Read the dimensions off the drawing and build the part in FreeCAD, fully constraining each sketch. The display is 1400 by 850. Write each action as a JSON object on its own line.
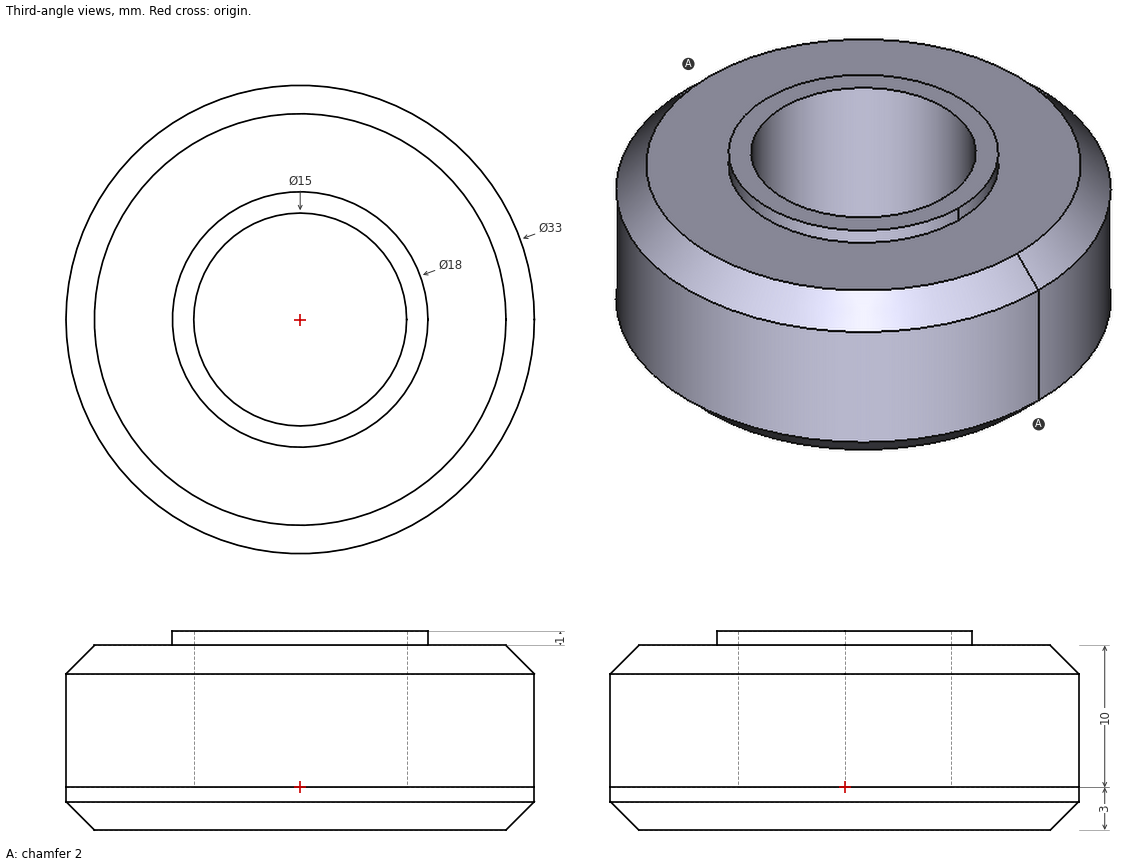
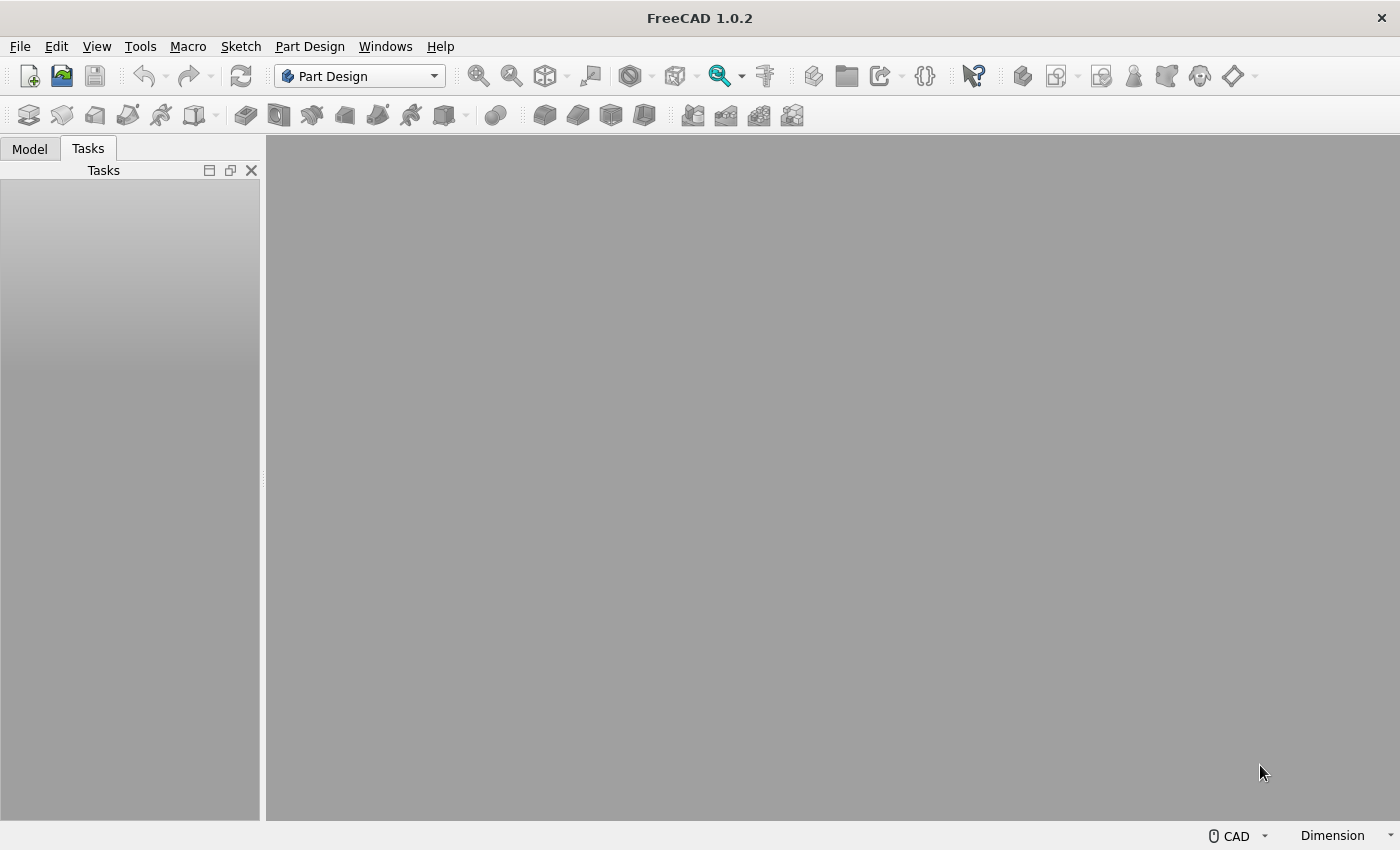
{"action": "key", "text": "ctrl+n"}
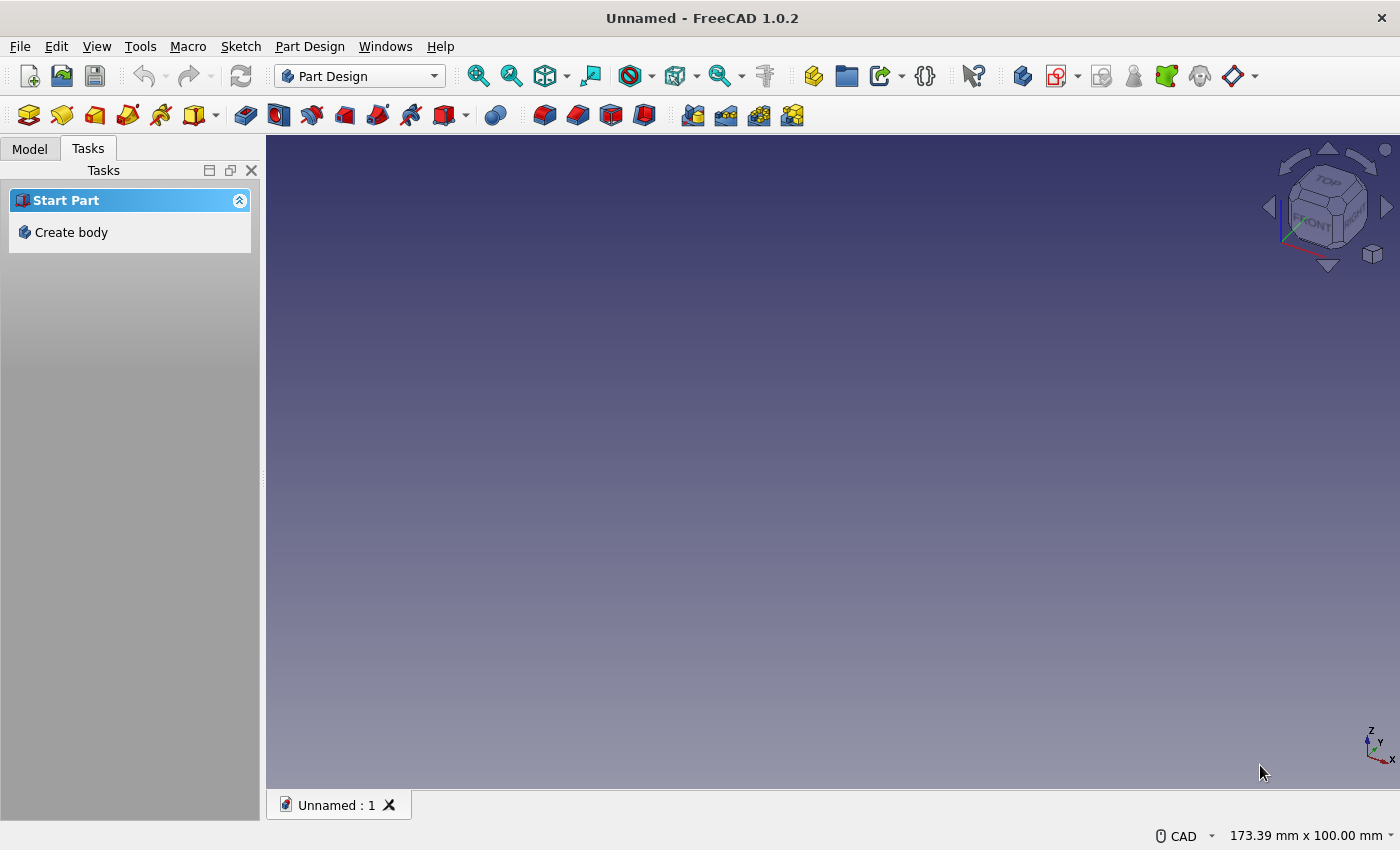
{"action": "left_click", "coordinate": [1056, 76]}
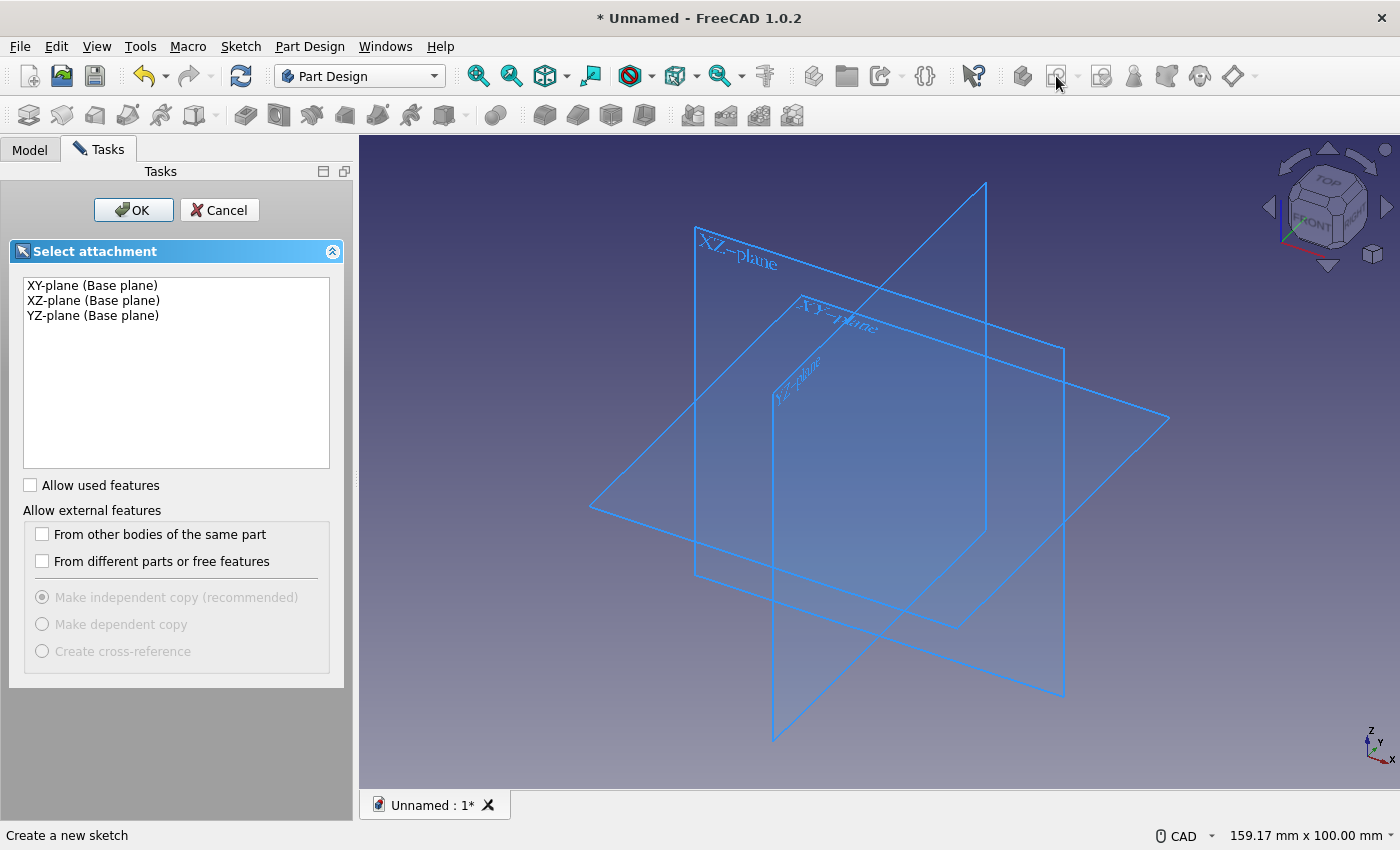
{"action": "left_click", "coordinate": [84, 286]}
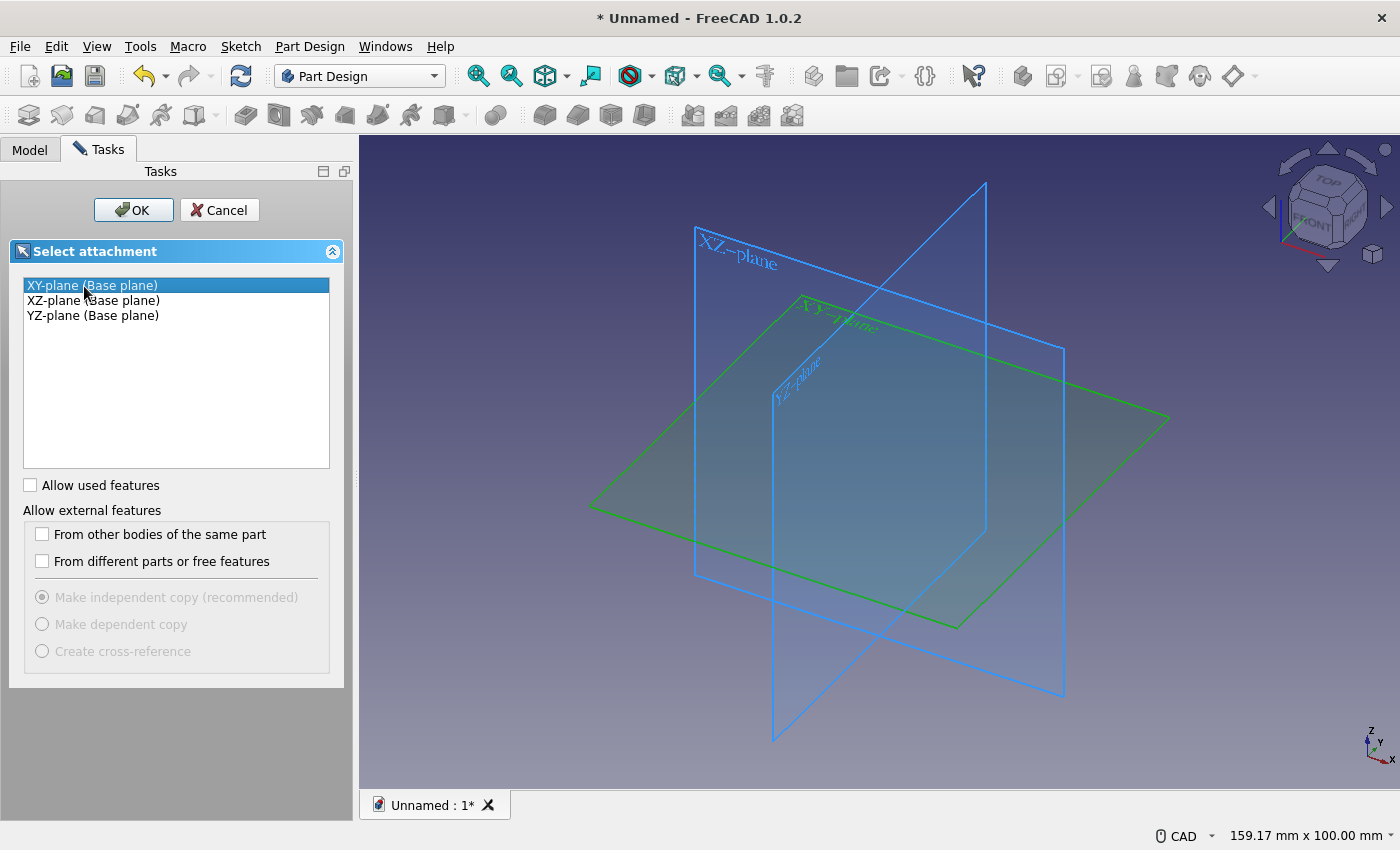
{"action": "left_click", "coordinate": [134, 210]}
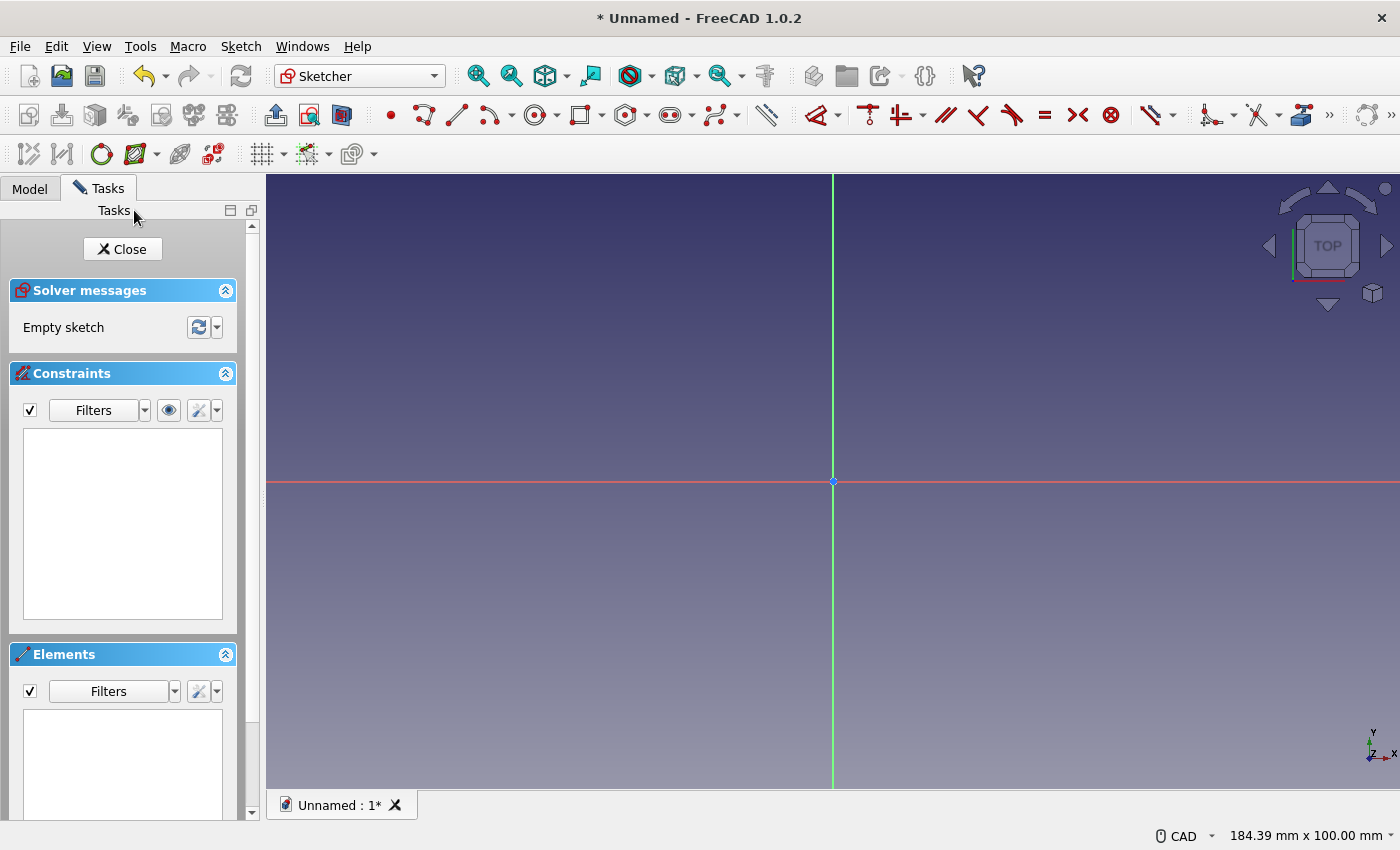
{"action": "scroll", "coordinate": [916, 481], "scroll_direction": "up", "scroll_amount": 3}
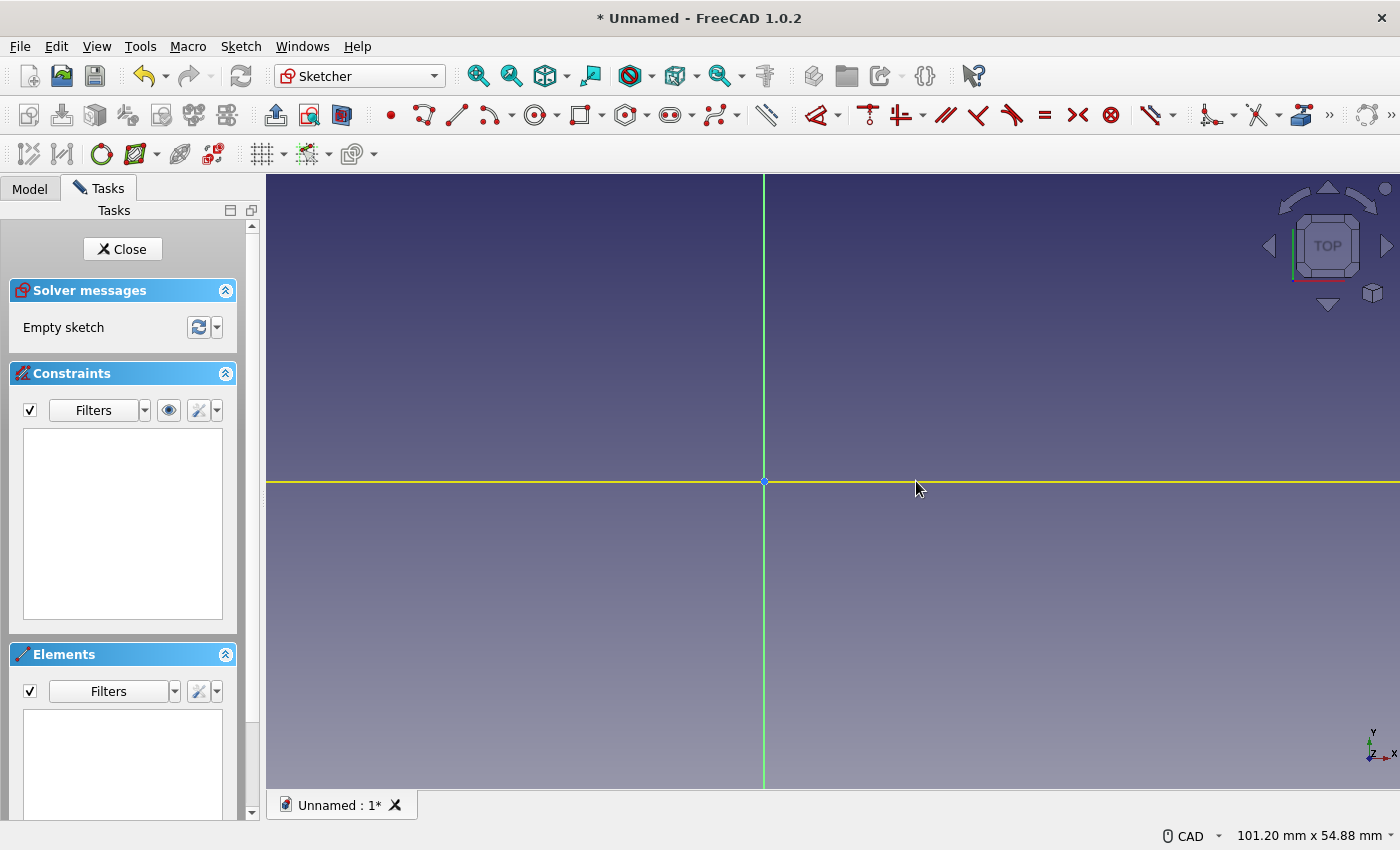
{"action": "key", "text": "g c"}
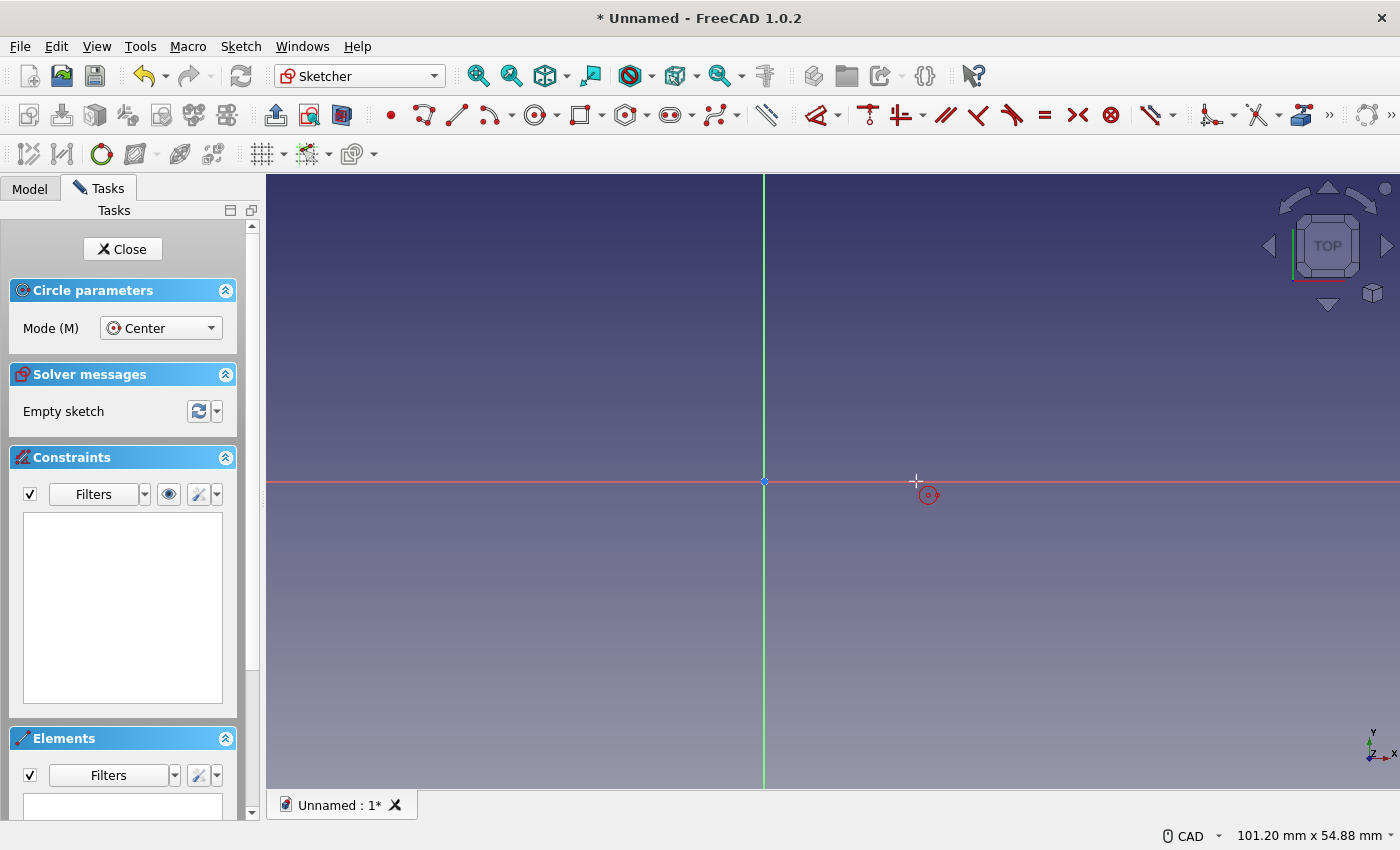
{"action": "left_click", "coordinate": [764, 482]}
{"action": "mouse_move", "coordinate": [895, 351]}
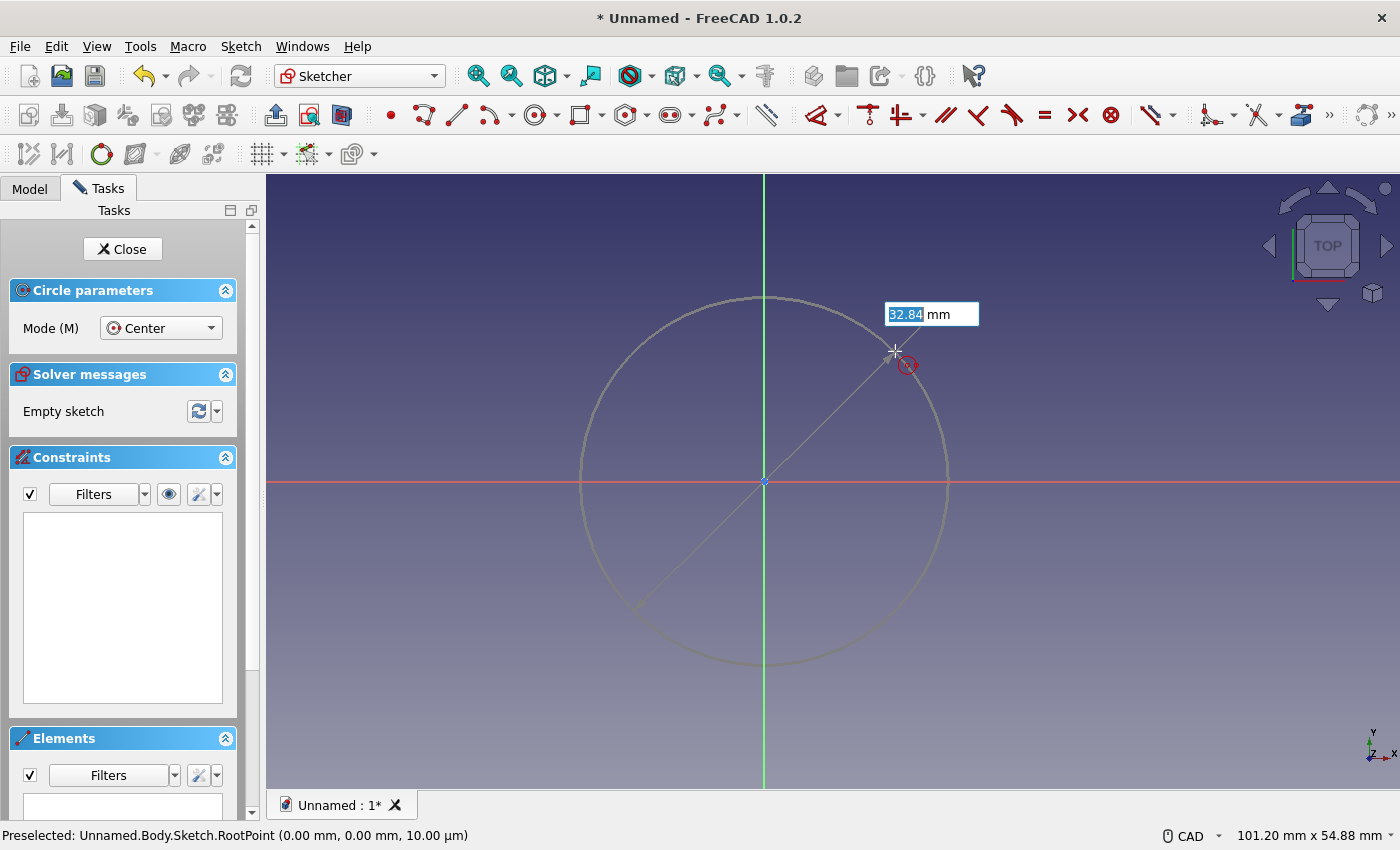
{"action": "type", "text": "33"}
{"action": "key", "text": "Return"}